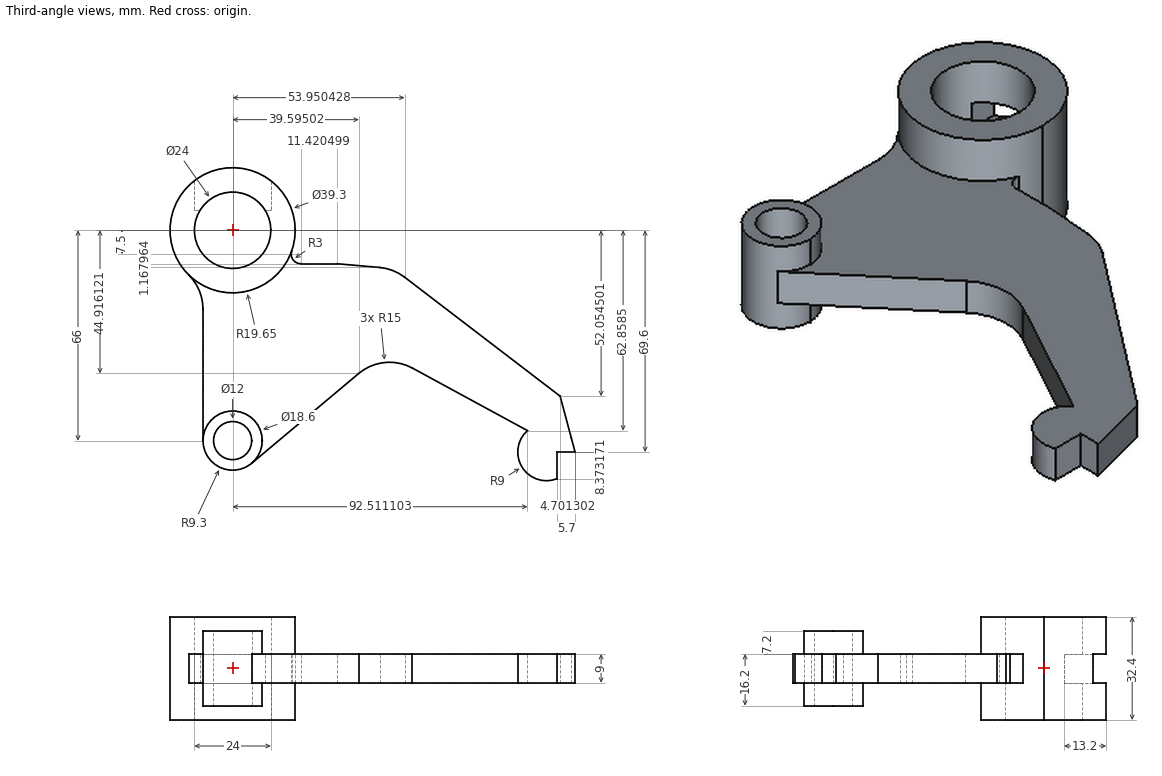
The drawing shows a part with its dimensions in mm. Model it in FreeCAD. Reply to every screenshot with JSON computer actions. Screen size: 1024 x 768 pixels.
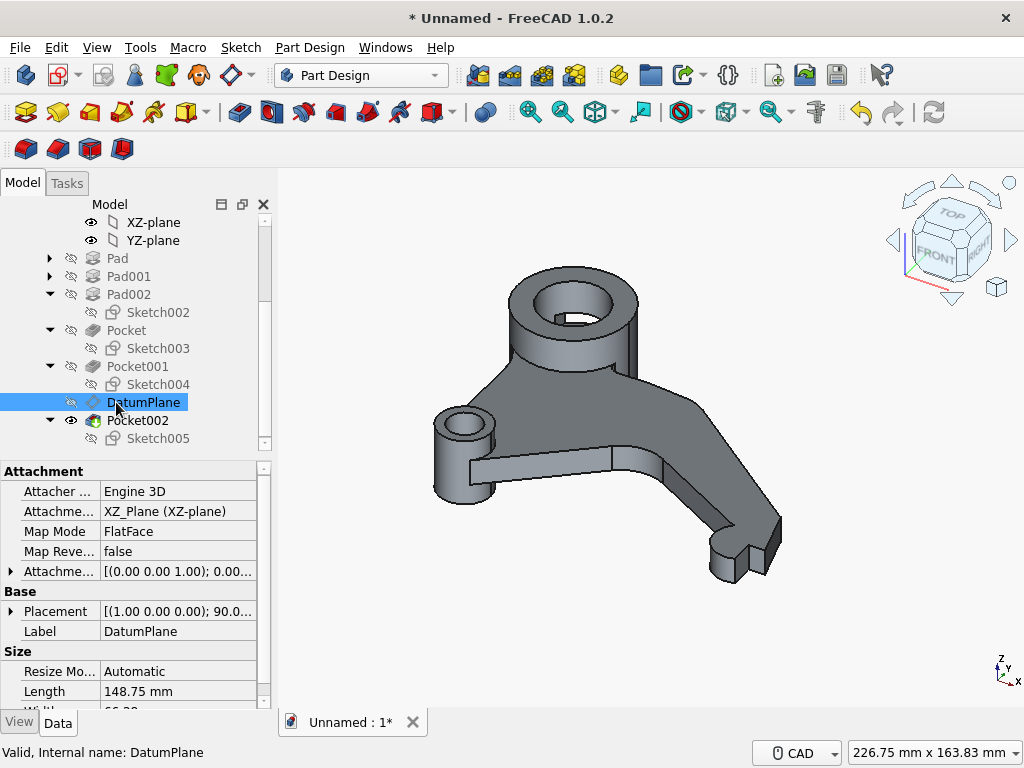
{"action": "key", "text": "0"}